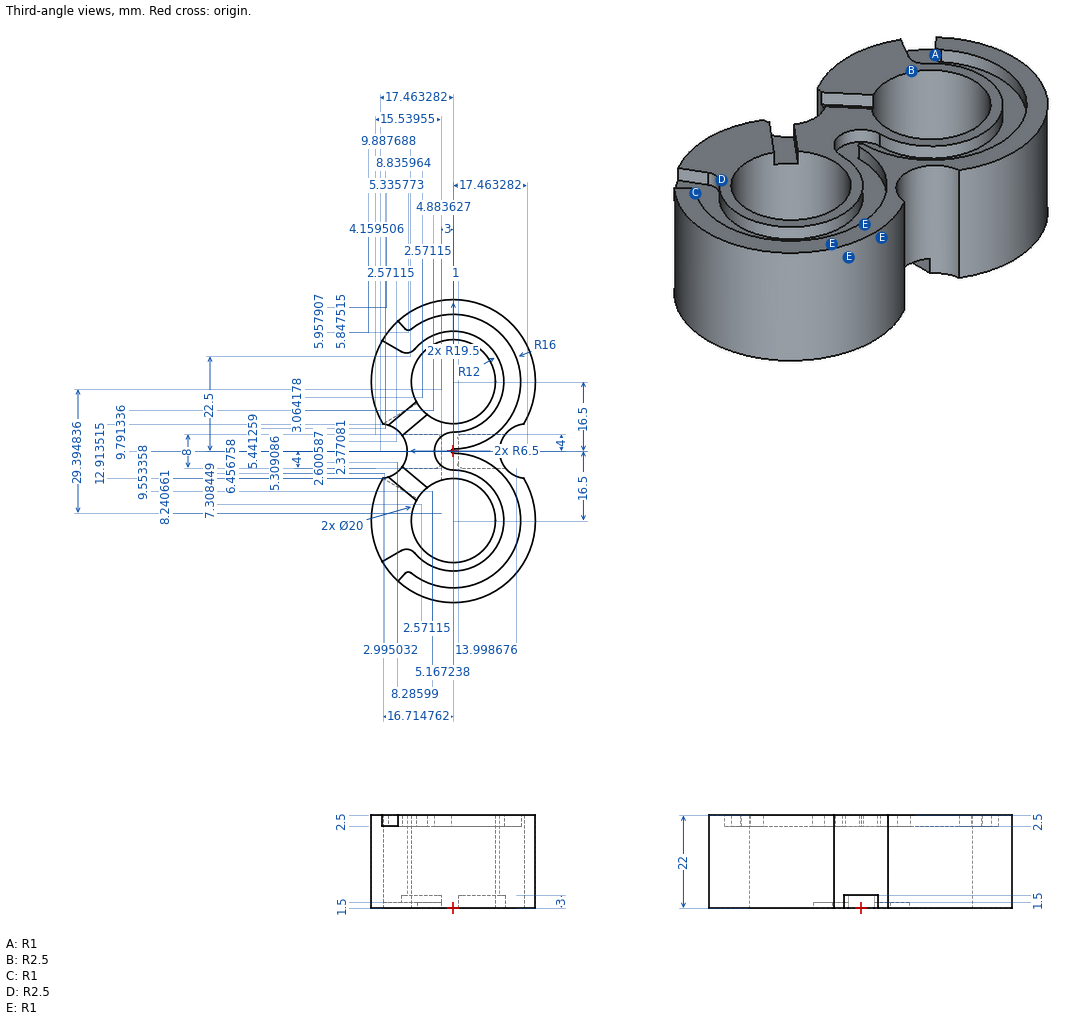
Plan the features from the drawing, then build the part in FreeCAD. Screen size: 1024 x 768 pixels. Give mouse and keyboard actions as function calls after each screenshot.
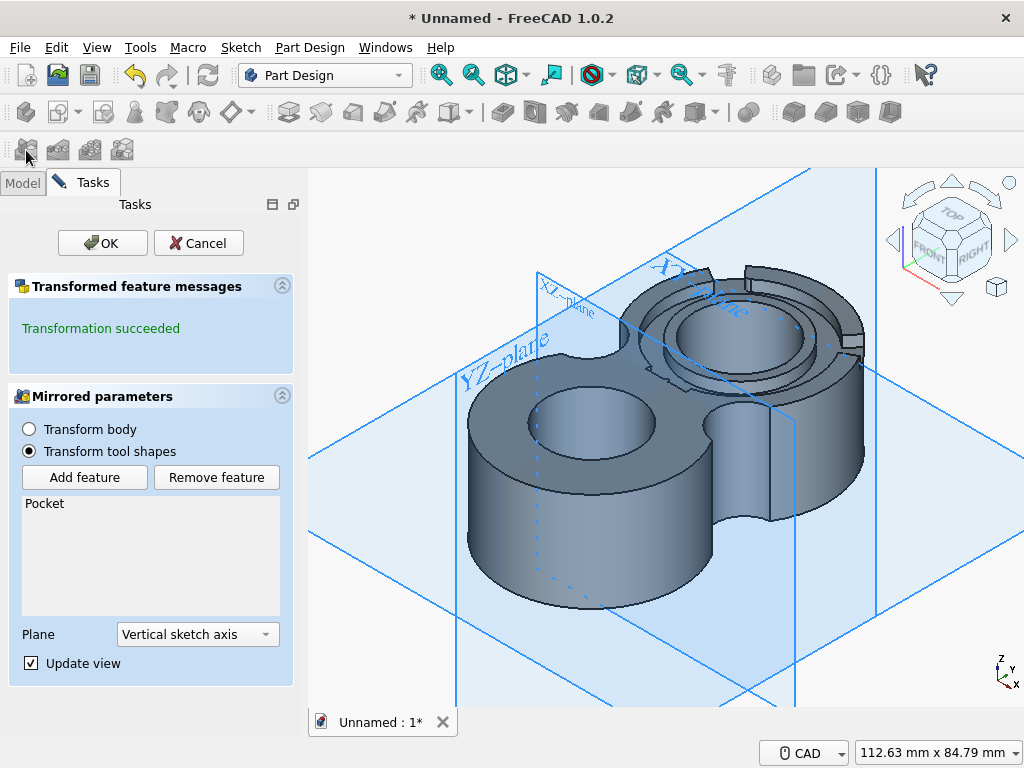
click(198, 634)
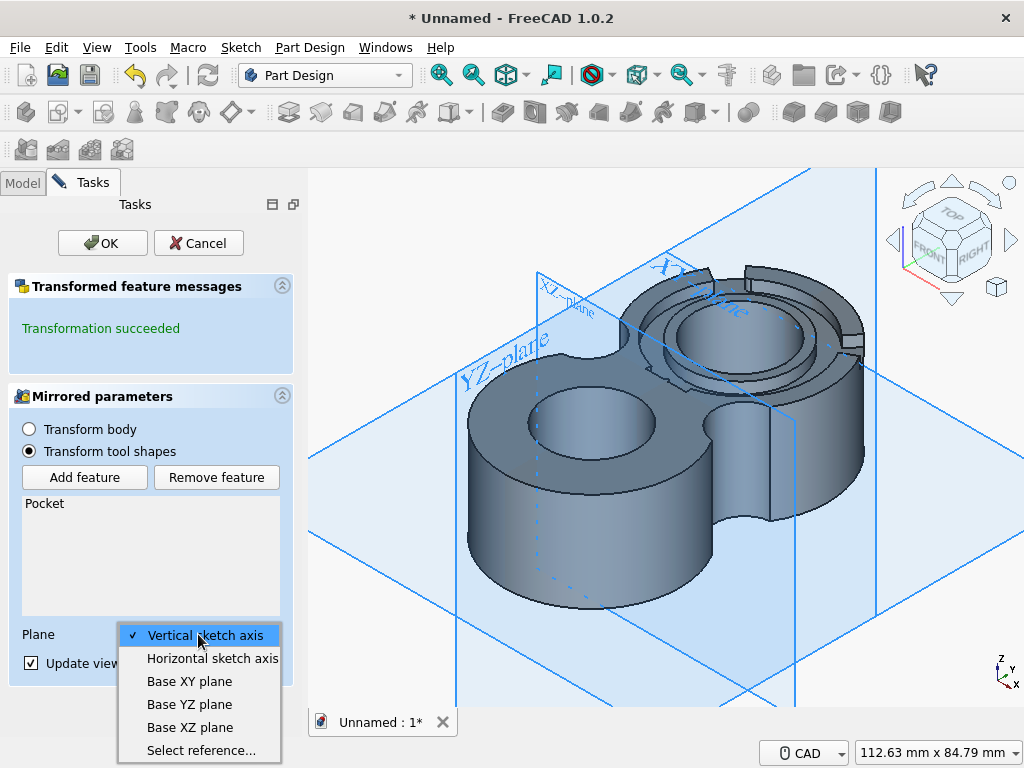
click(198, 728)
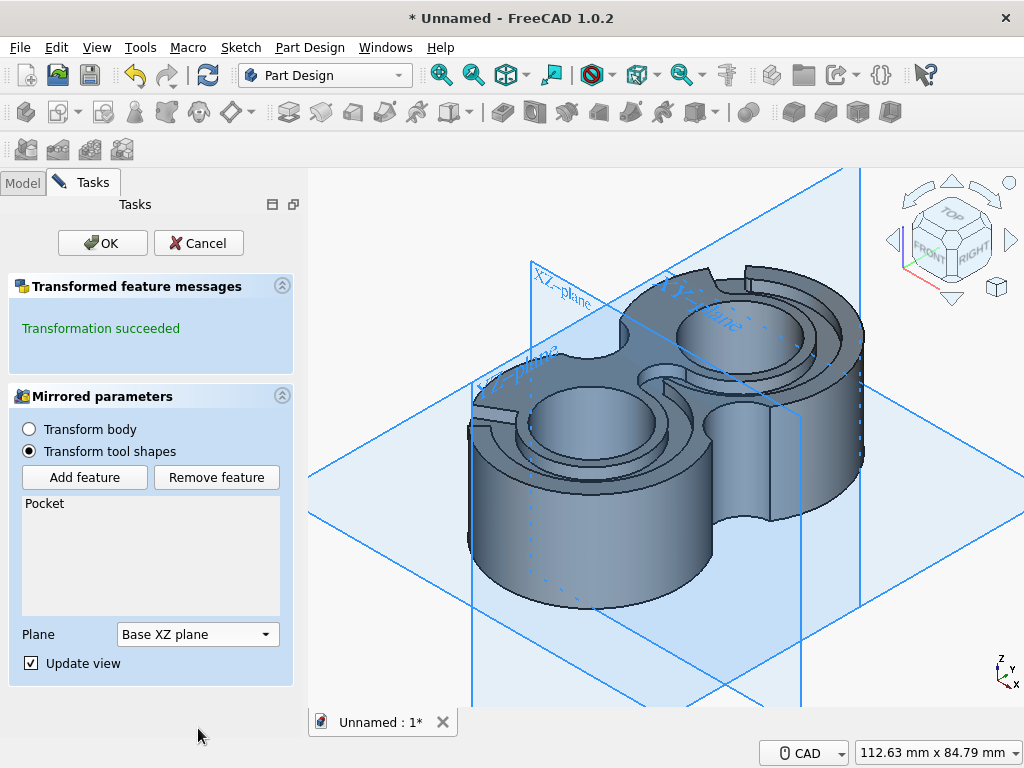
click(103, 243)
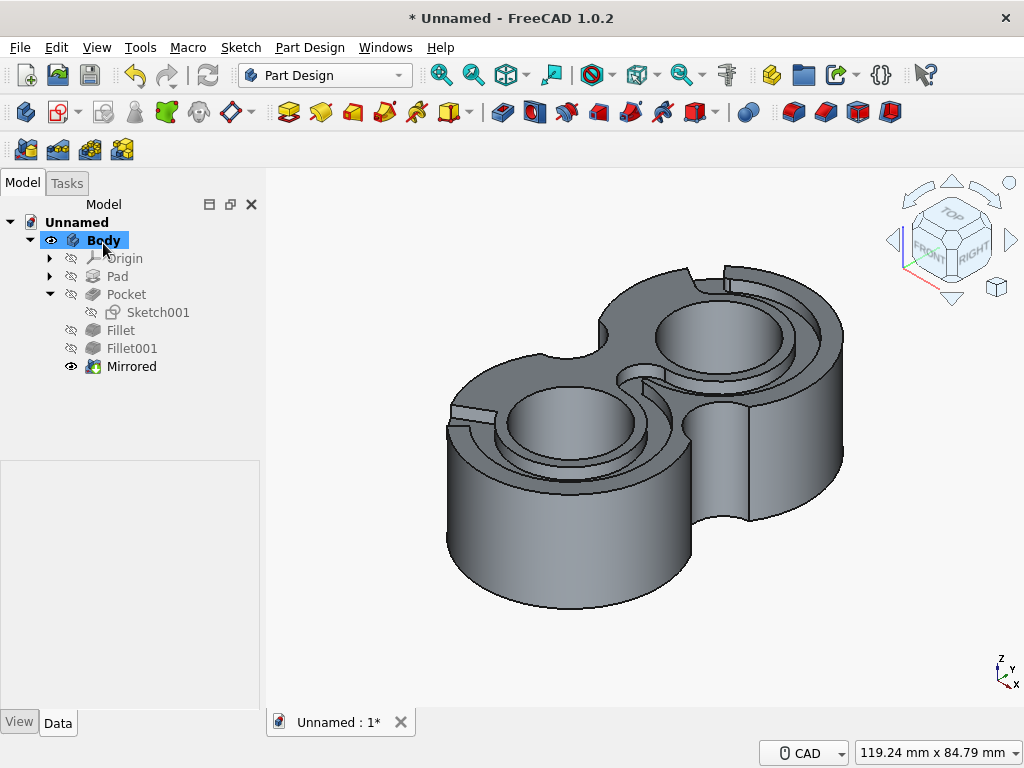
scroll(469, 431, up, 5)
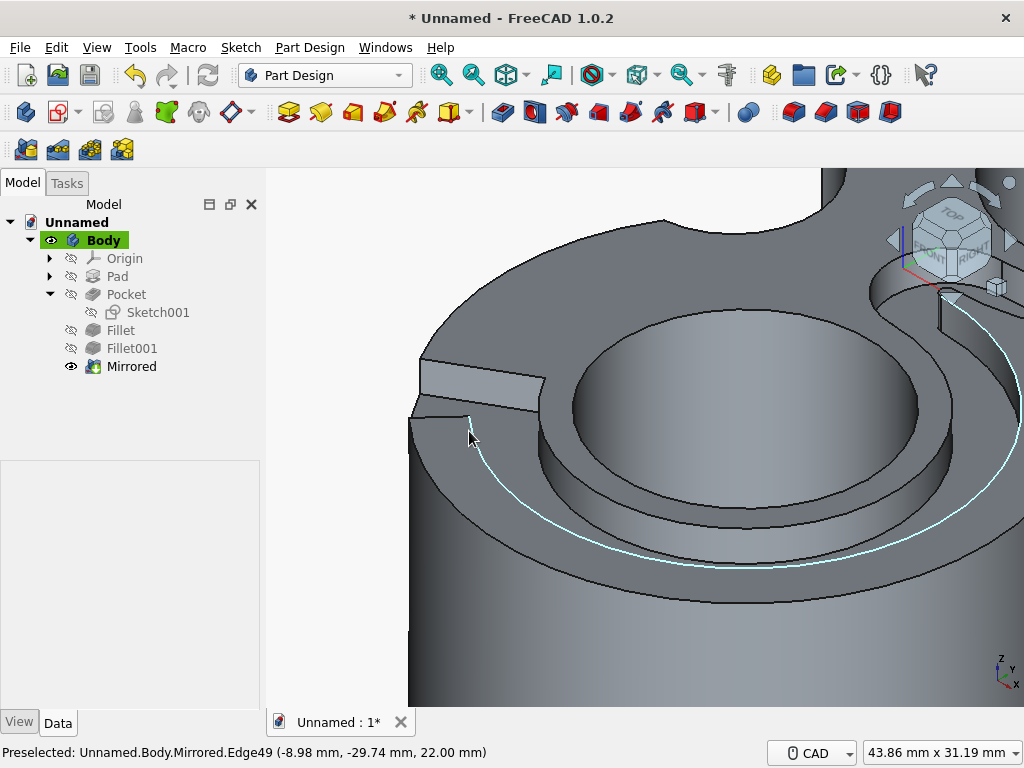
click(442, 76)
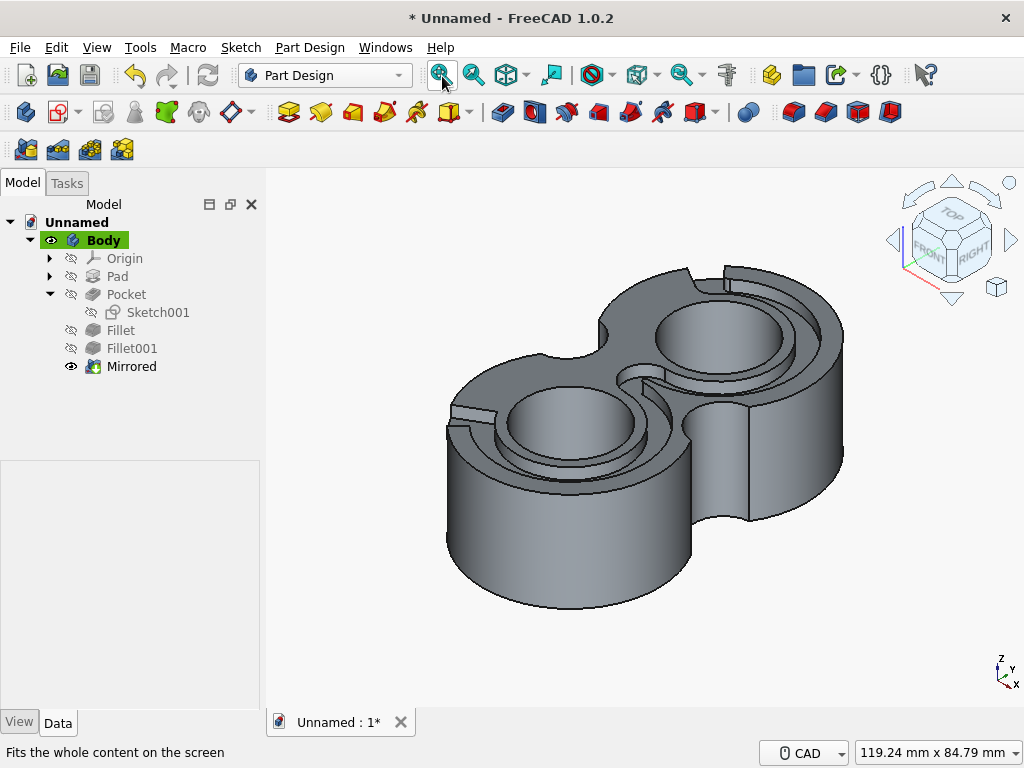
key(2)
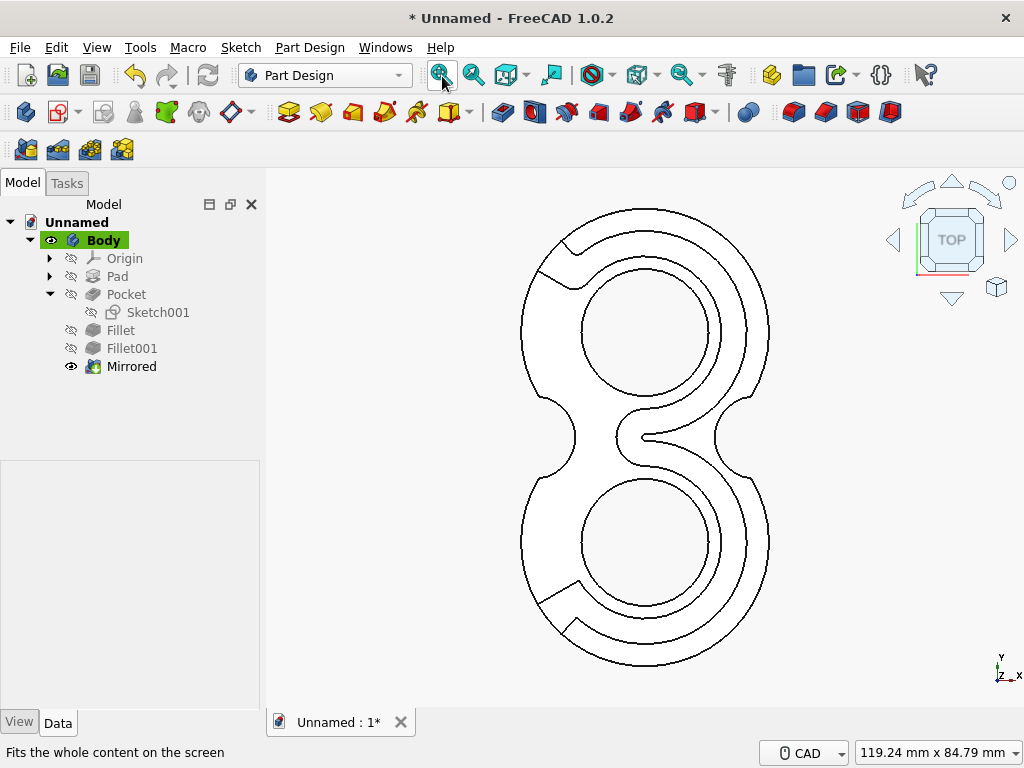
scroll(576, 617, up, 5)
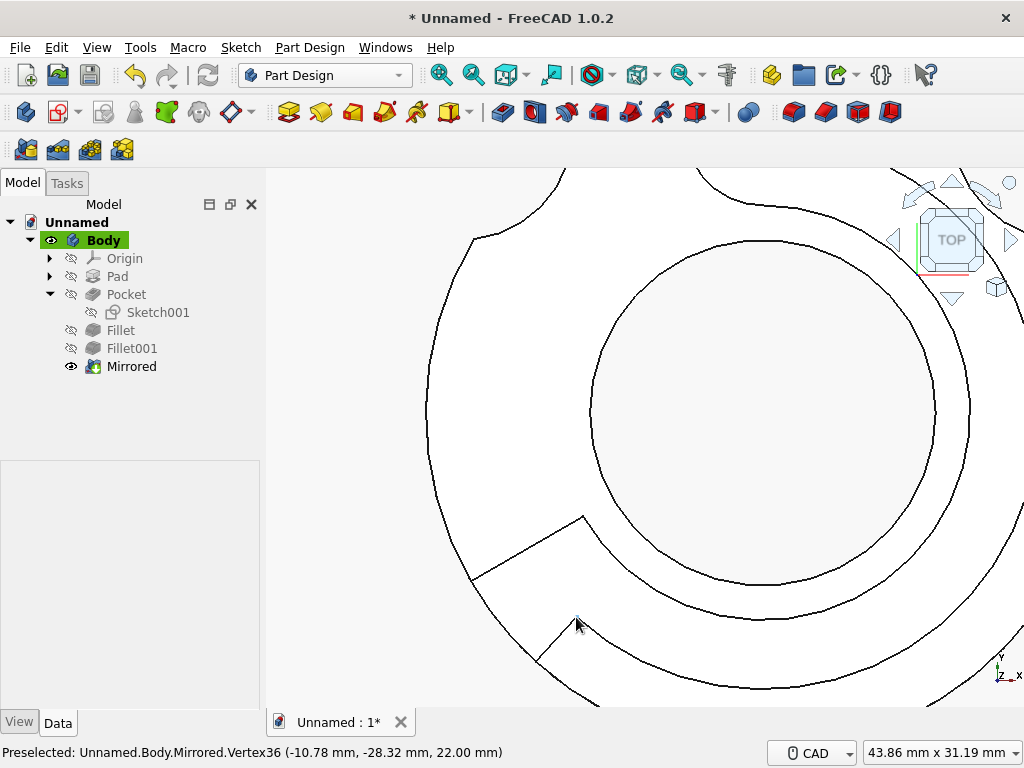
key(v)
key(f)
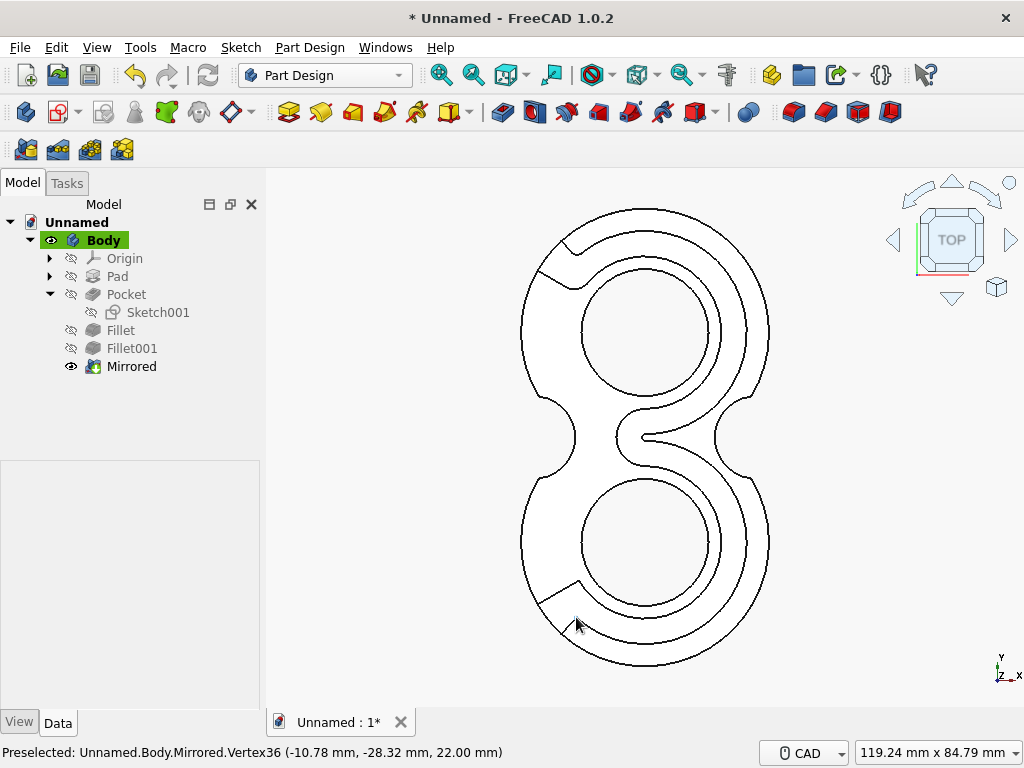
key(0)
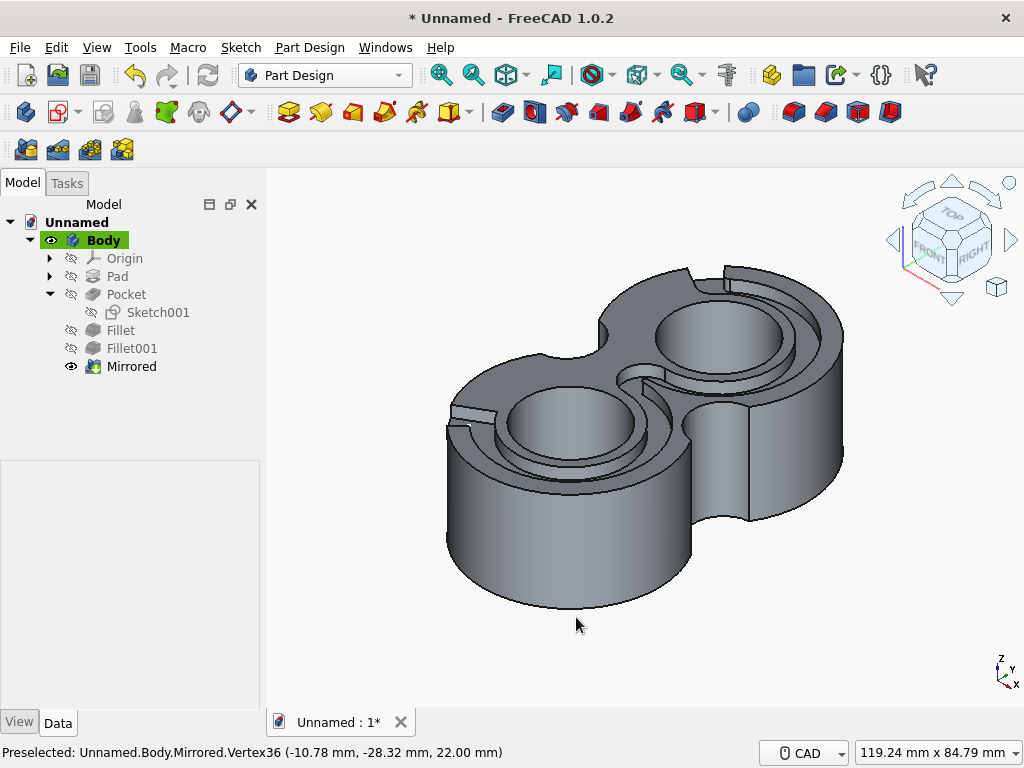
scroll(469, 431, up, 5)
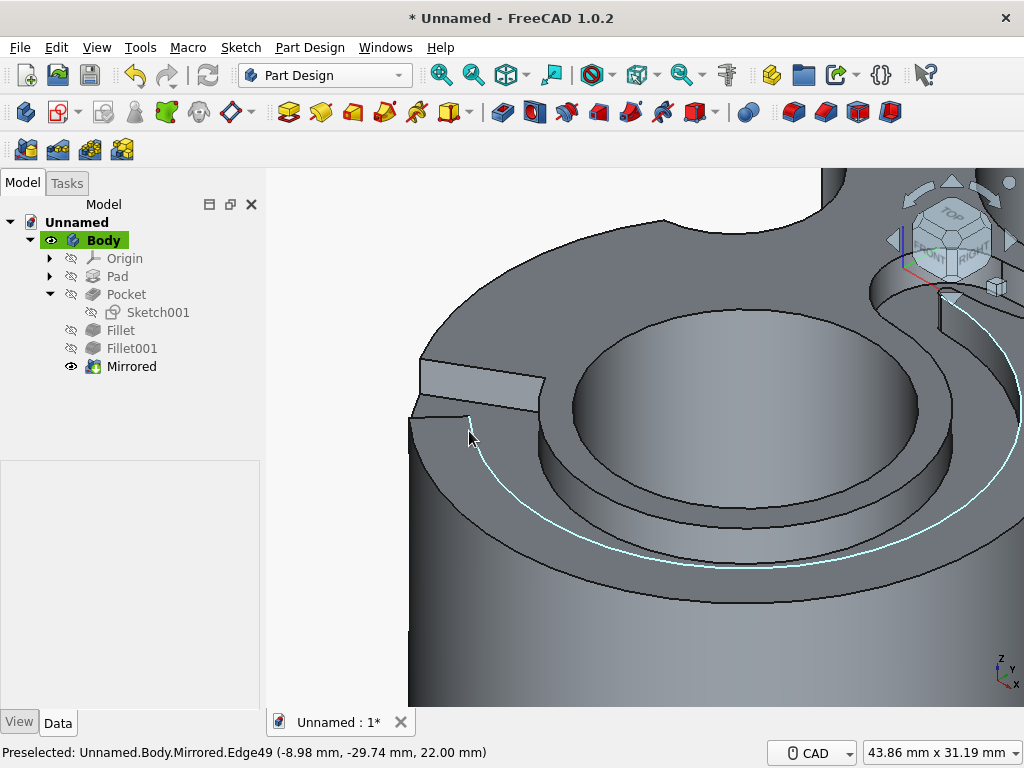
key(v)
key(f)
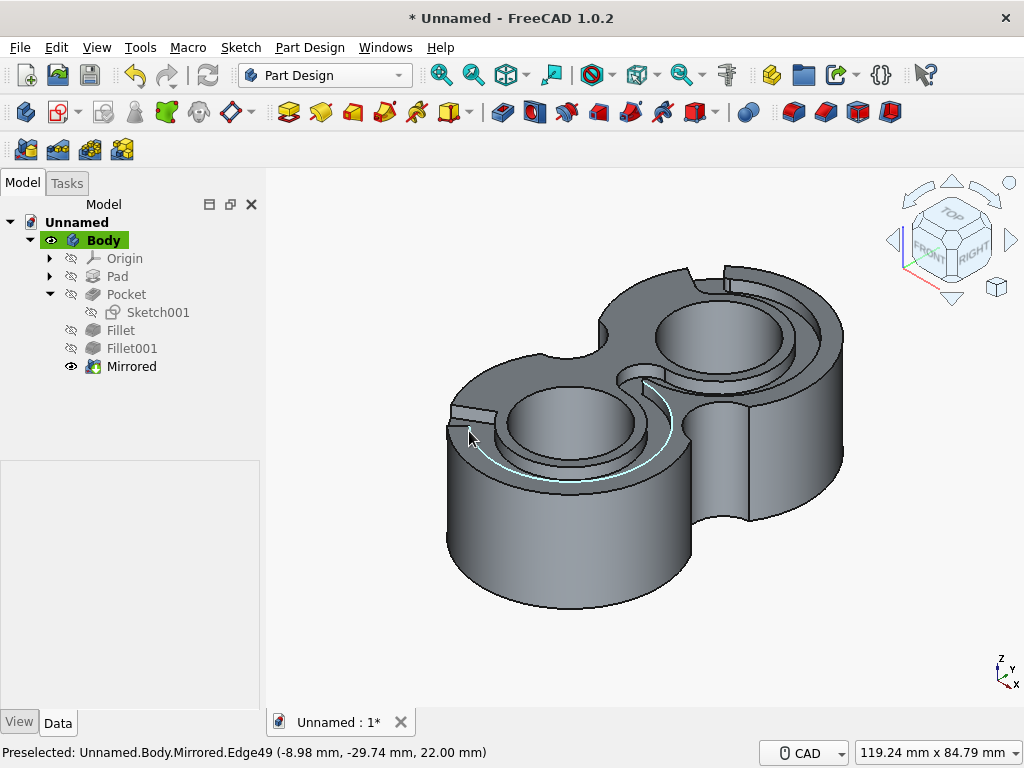
key(1)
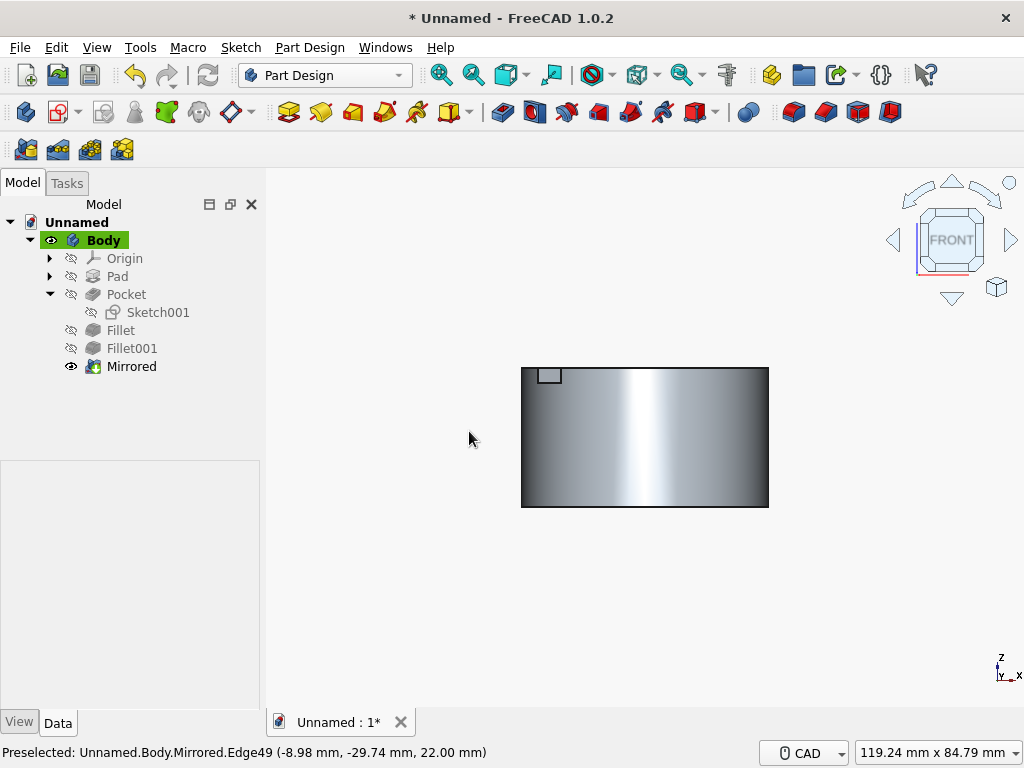
key(v)
key(f)